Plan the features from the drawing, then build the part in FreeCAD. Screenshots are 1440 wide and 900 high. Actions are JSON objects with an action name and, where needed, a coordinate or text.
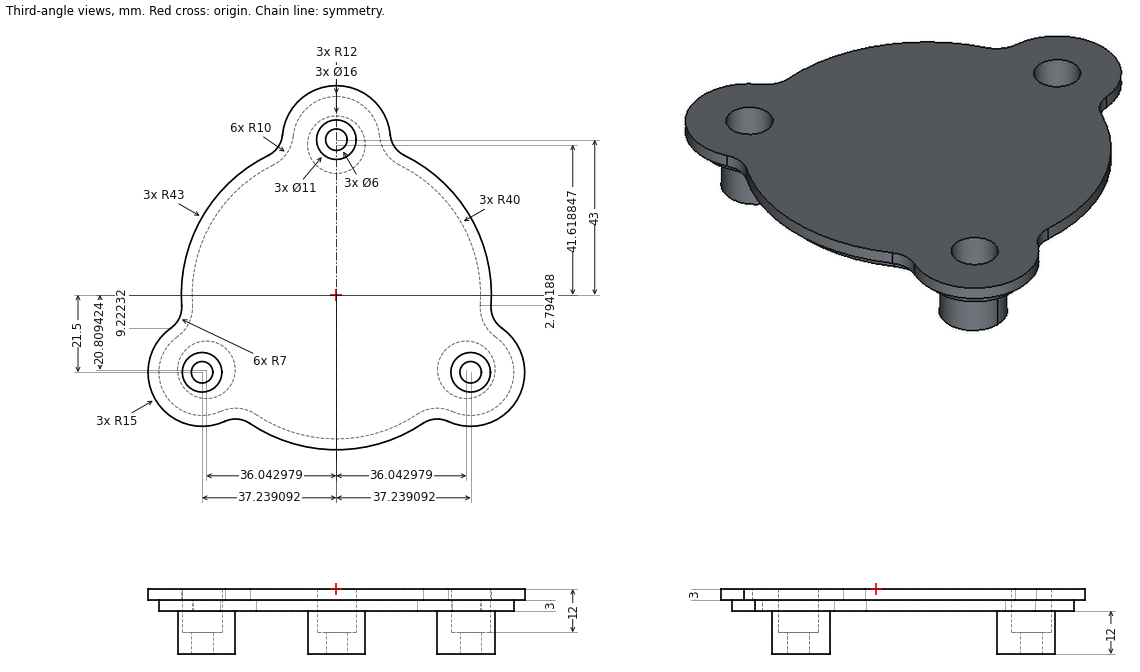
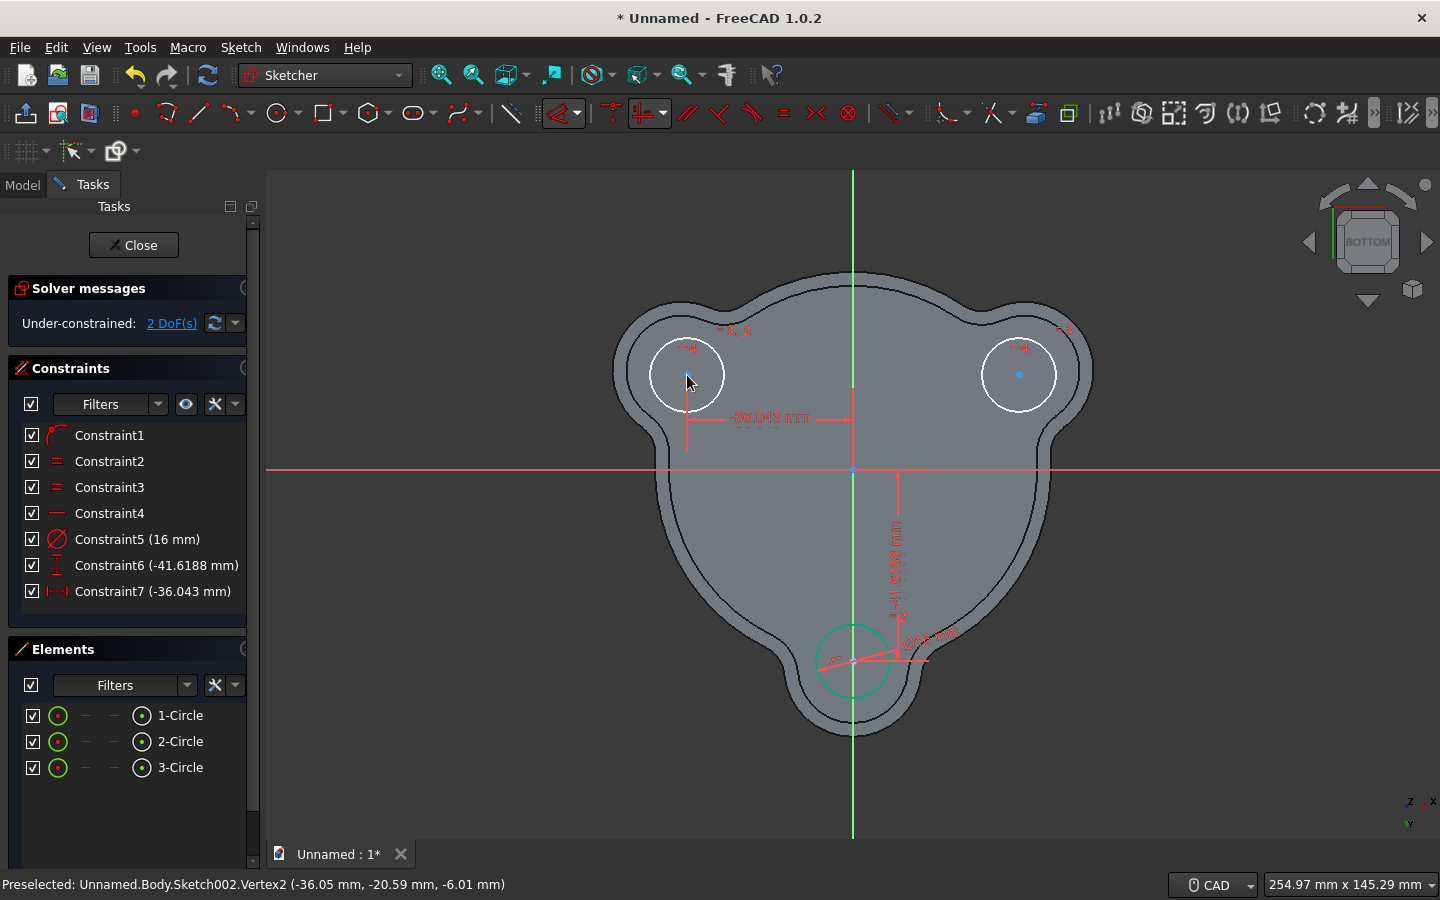
{"action": "left_click", "coordinate": [687, 375]}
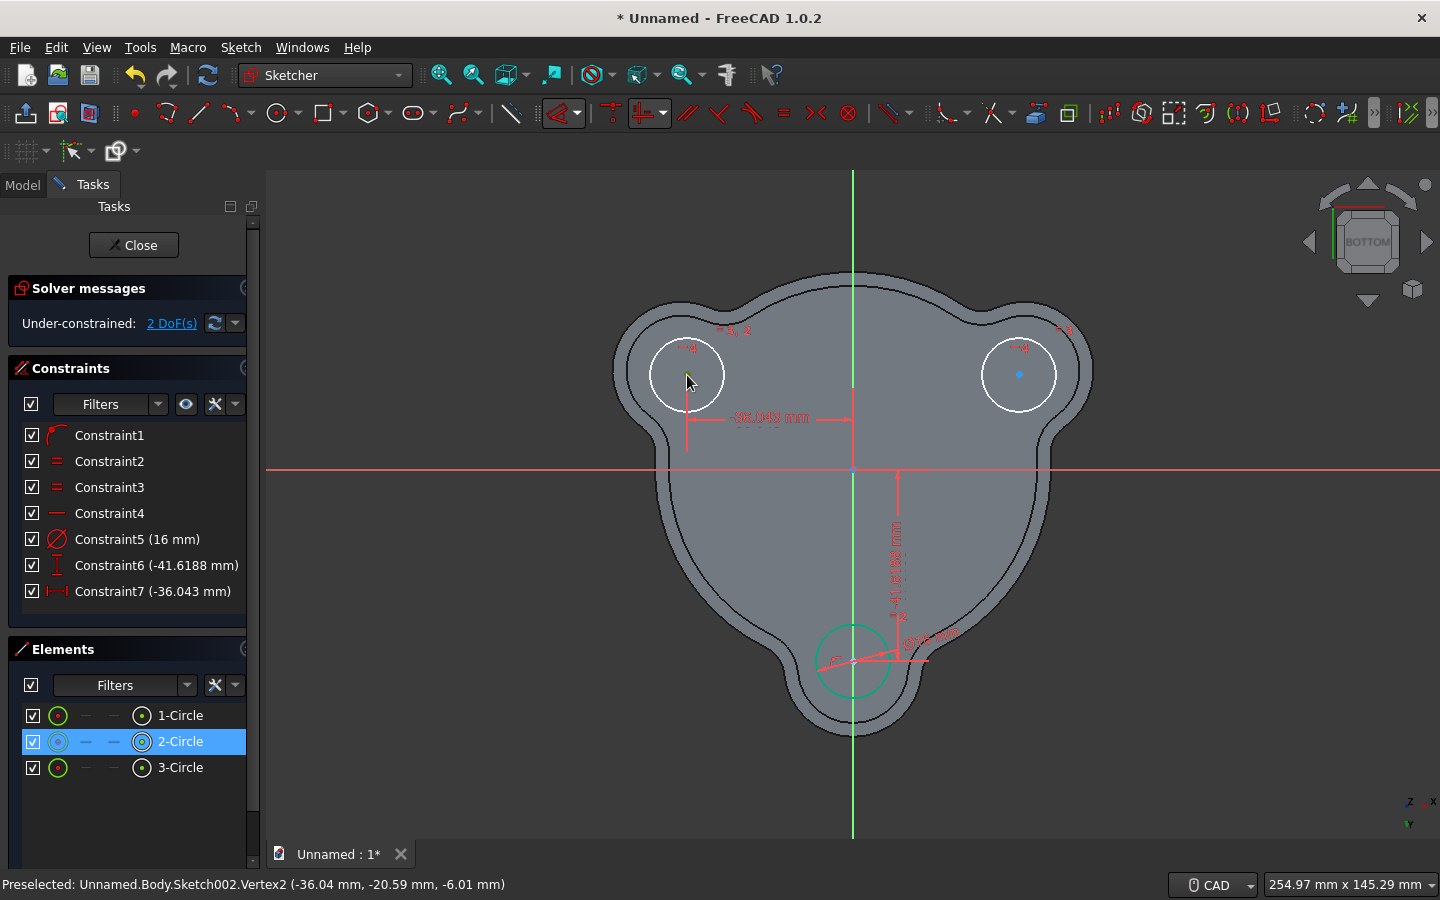
{"action": "key", "text": "i"}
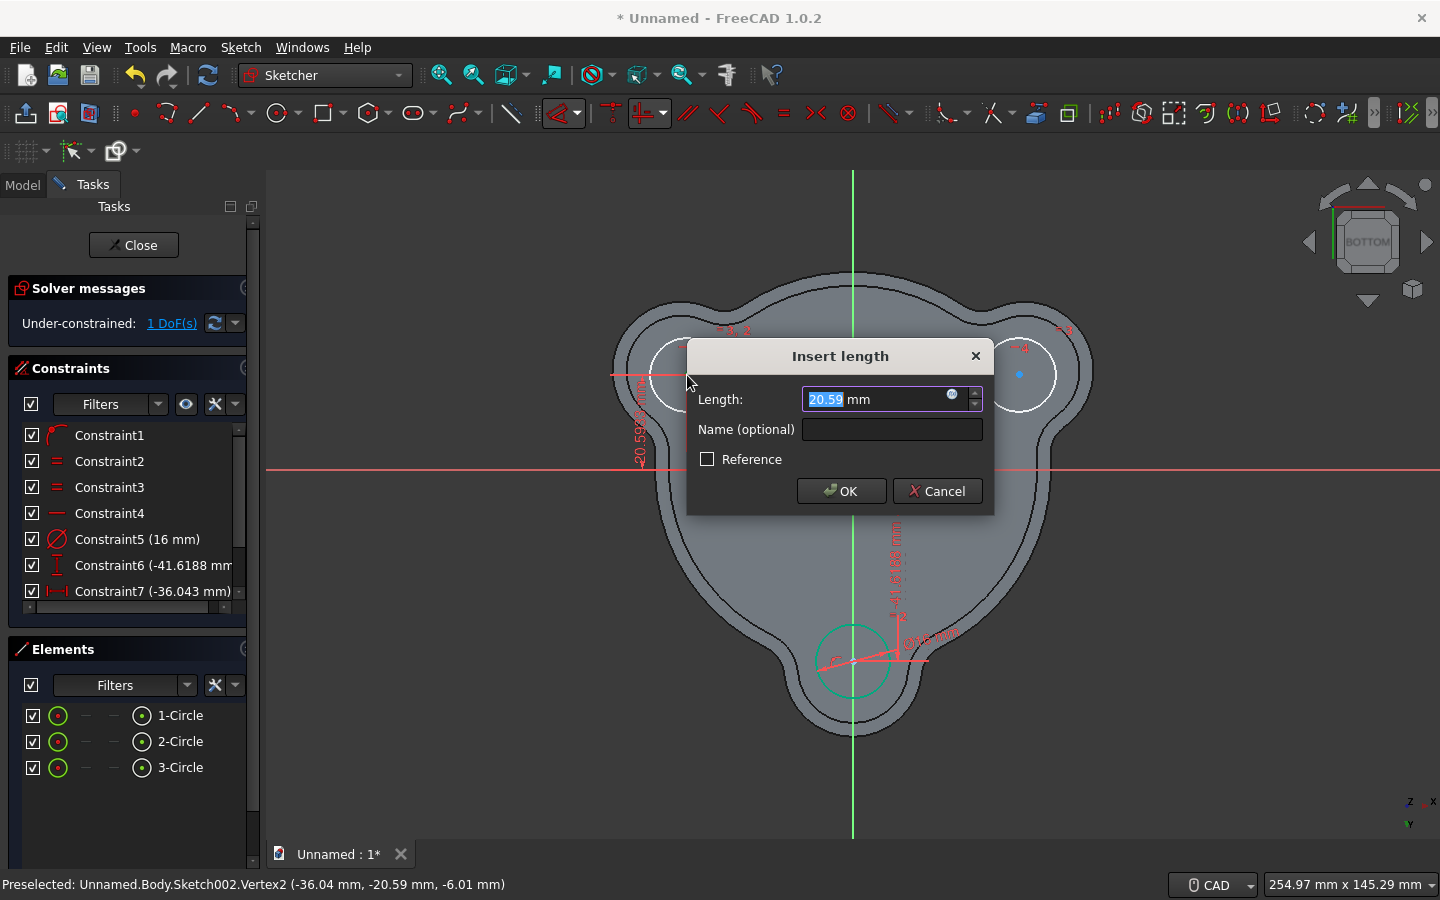
{"action": "type", "text": "20.809424"}
{"action": "key", "text": "Return"}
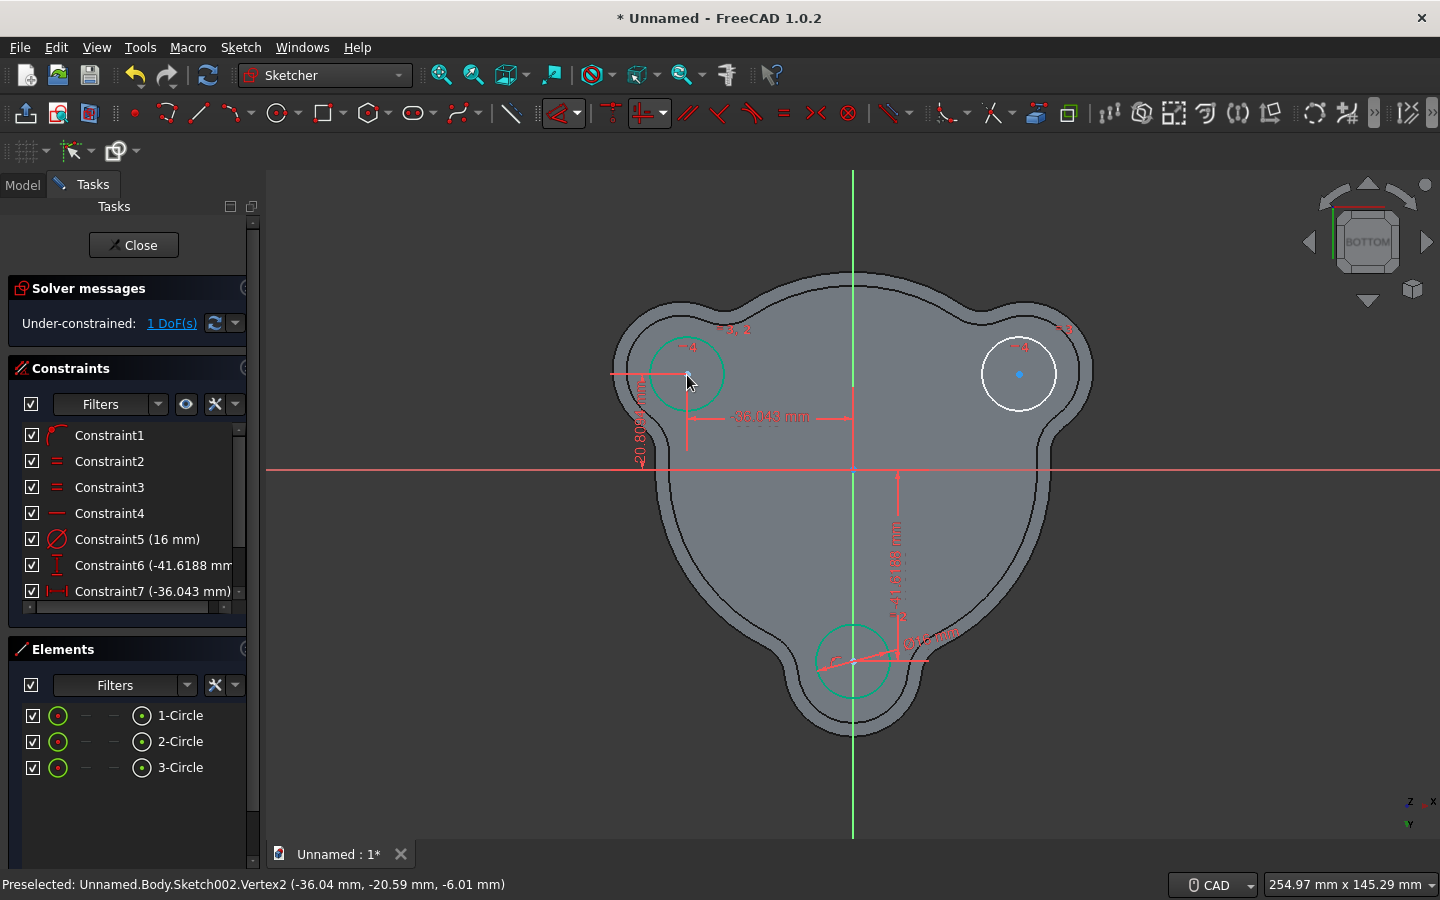
{"action": "left_click", "coordinate": [1019, 374]}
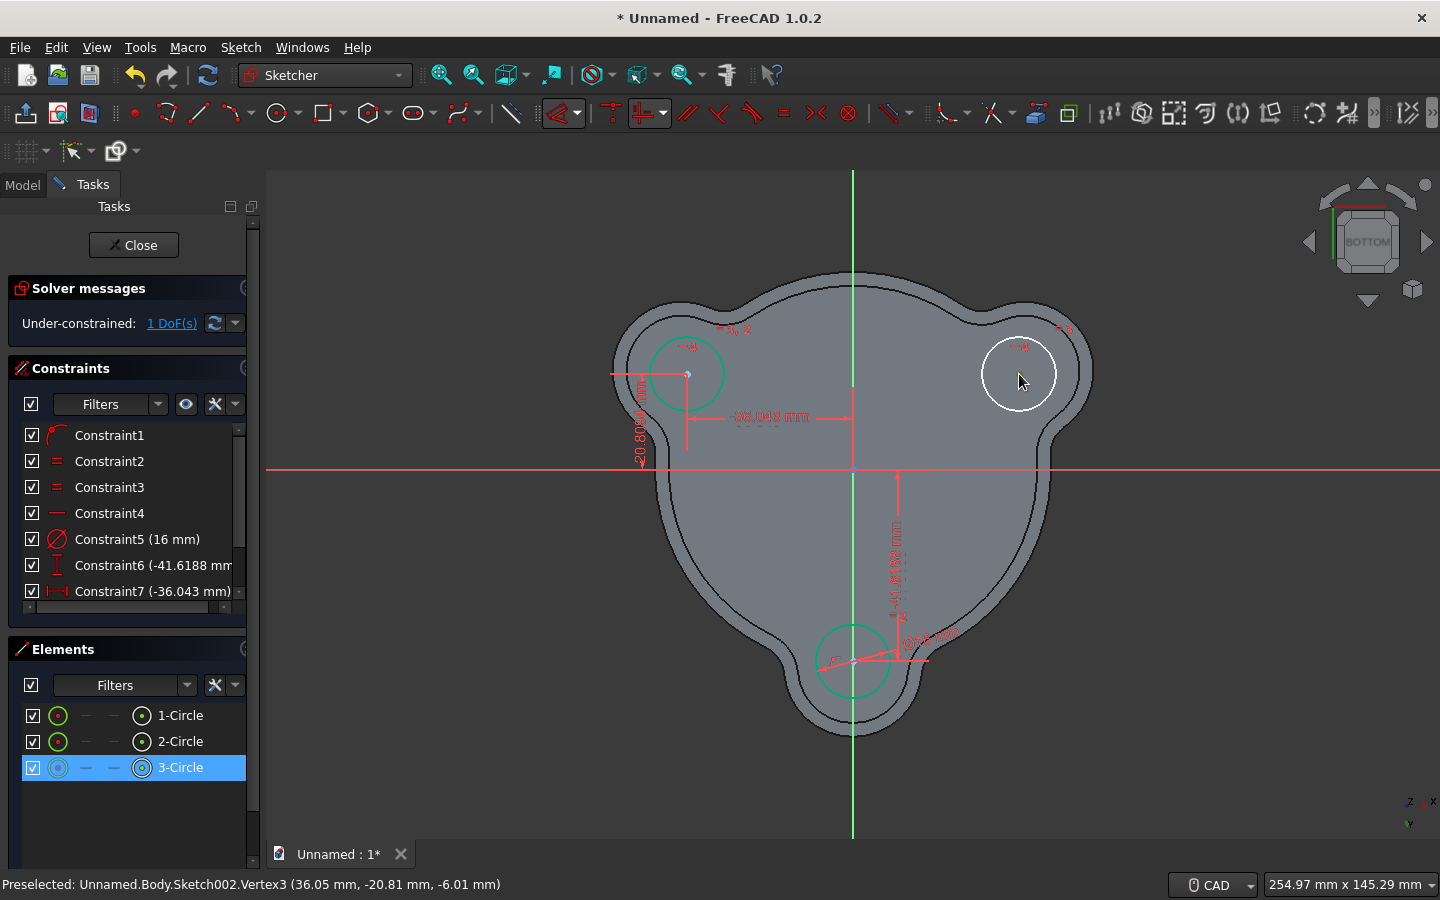
{"action": "left_click", "coordinate": [580, 114]}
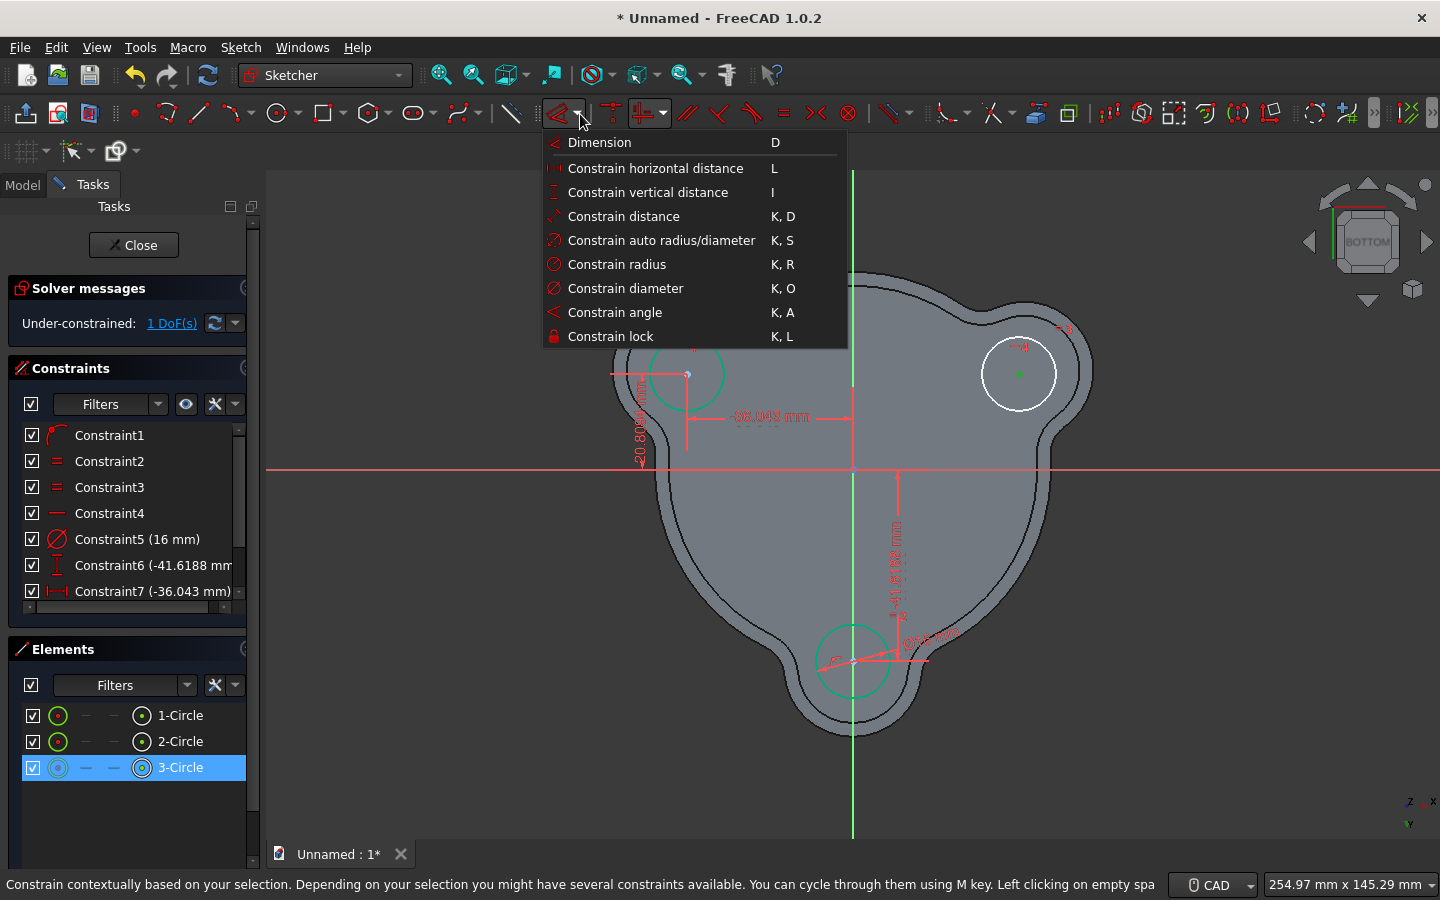
{"action": "left_click", "coordinate": [695, 168]}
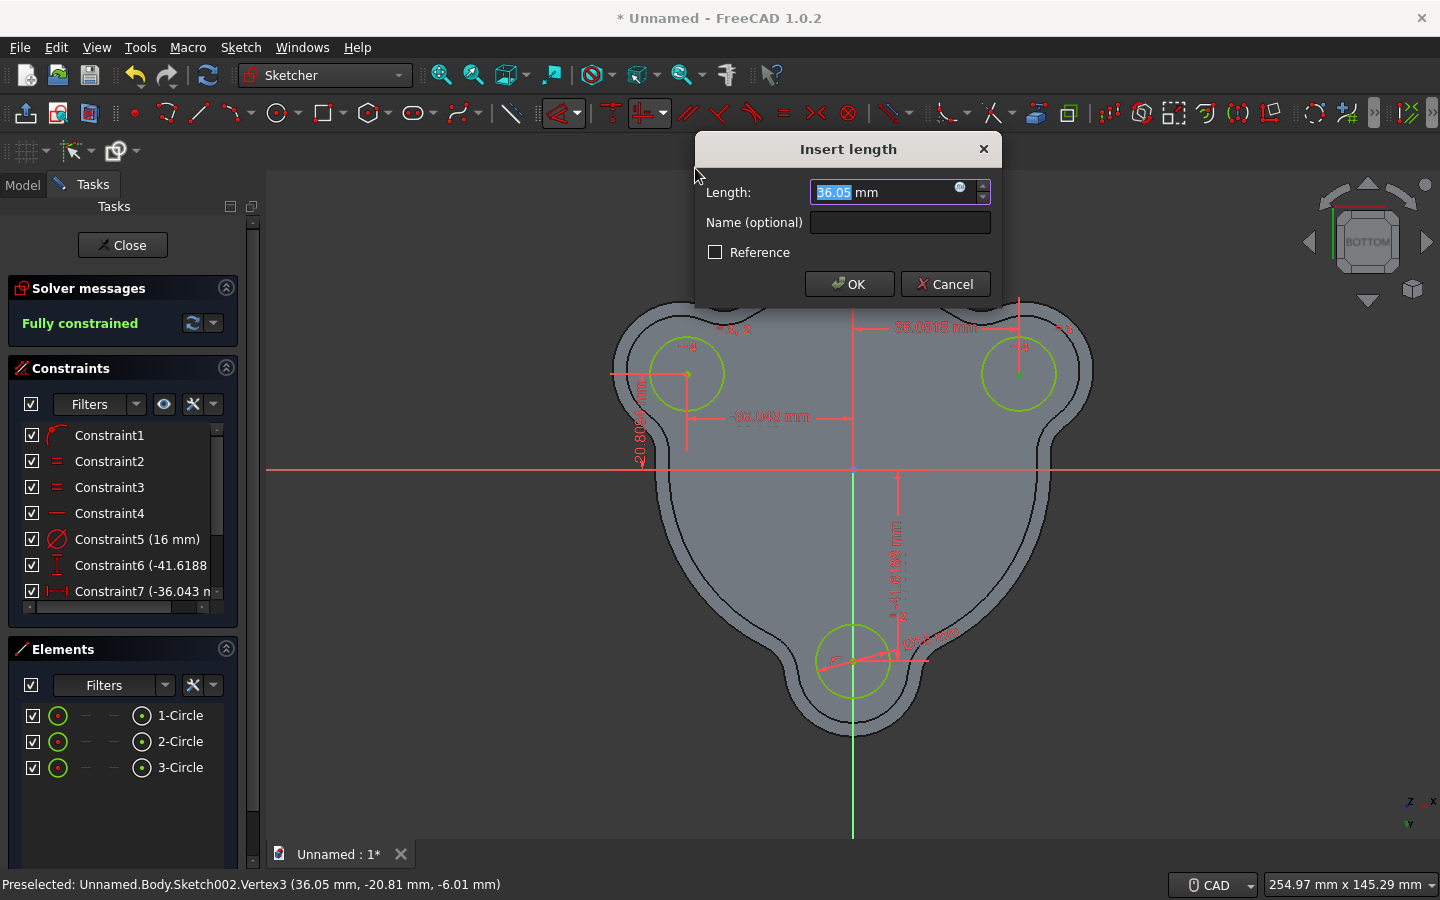
{"action": "type", "text": "36.042979"}
{"action": "key", "text": "Return"}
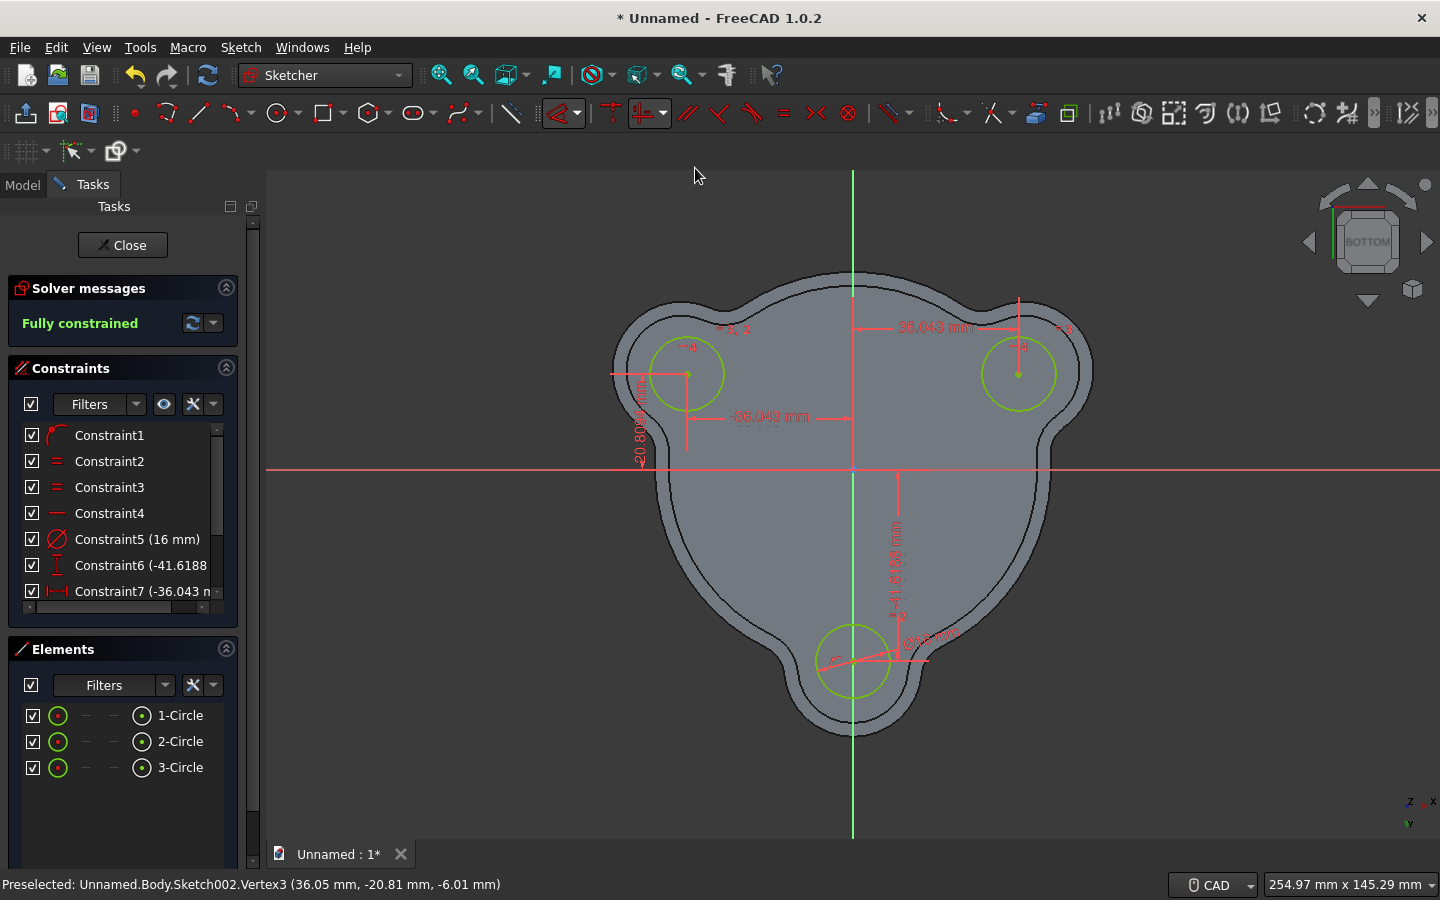
{"action": "left_click", "coordinate": [123, 245]}